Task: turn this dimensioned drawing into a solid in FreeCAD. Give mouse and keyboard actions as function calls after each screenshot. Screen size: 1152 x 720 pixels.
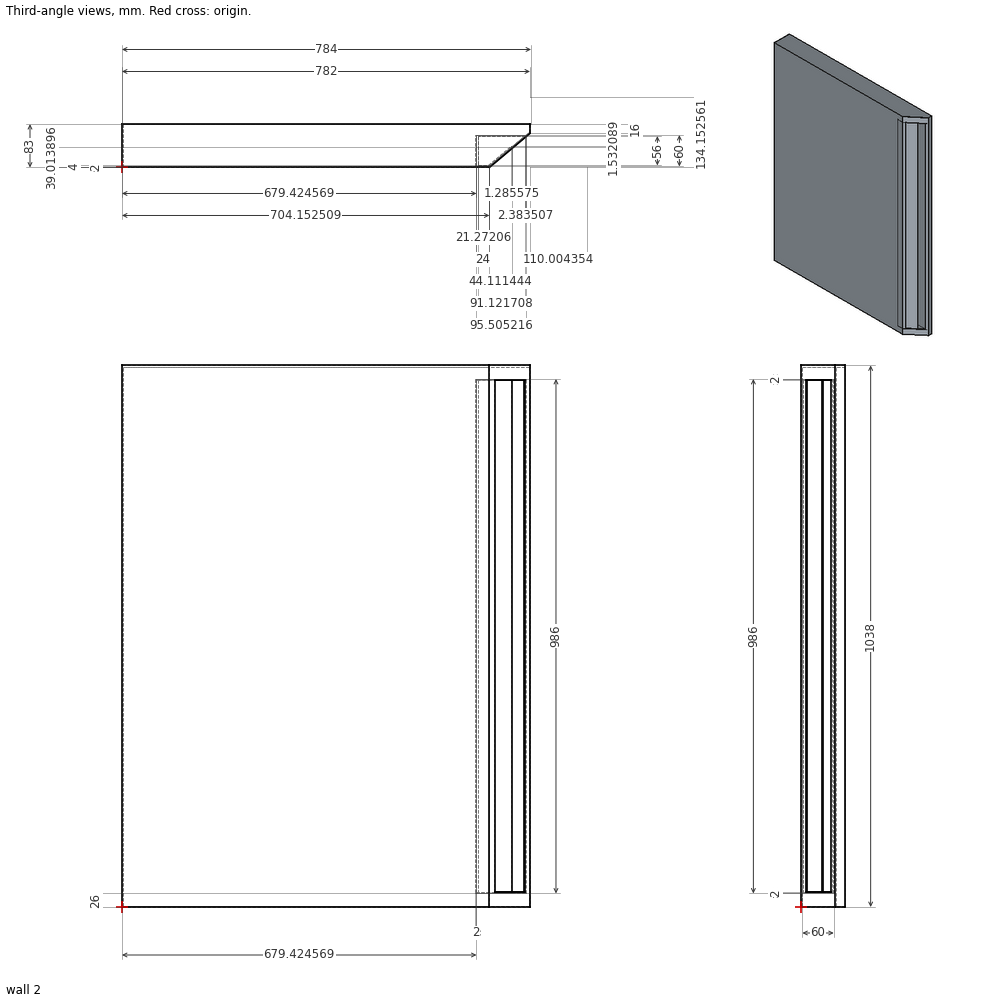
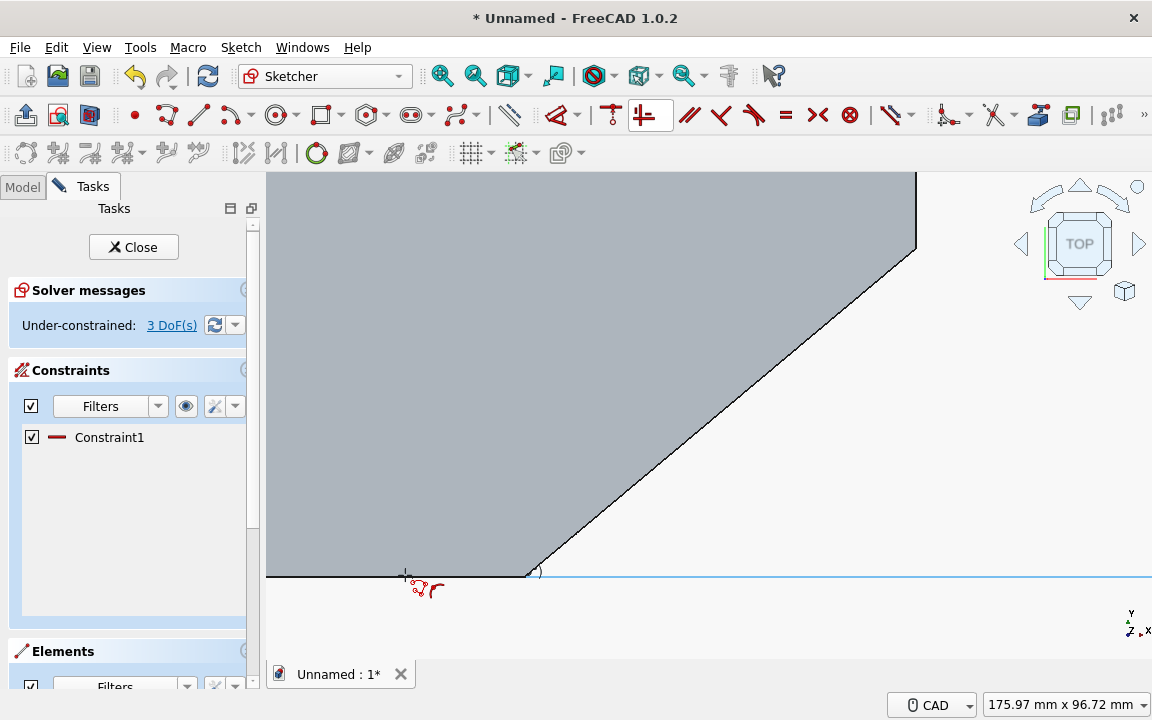
click(881, 265)
click(400, 265)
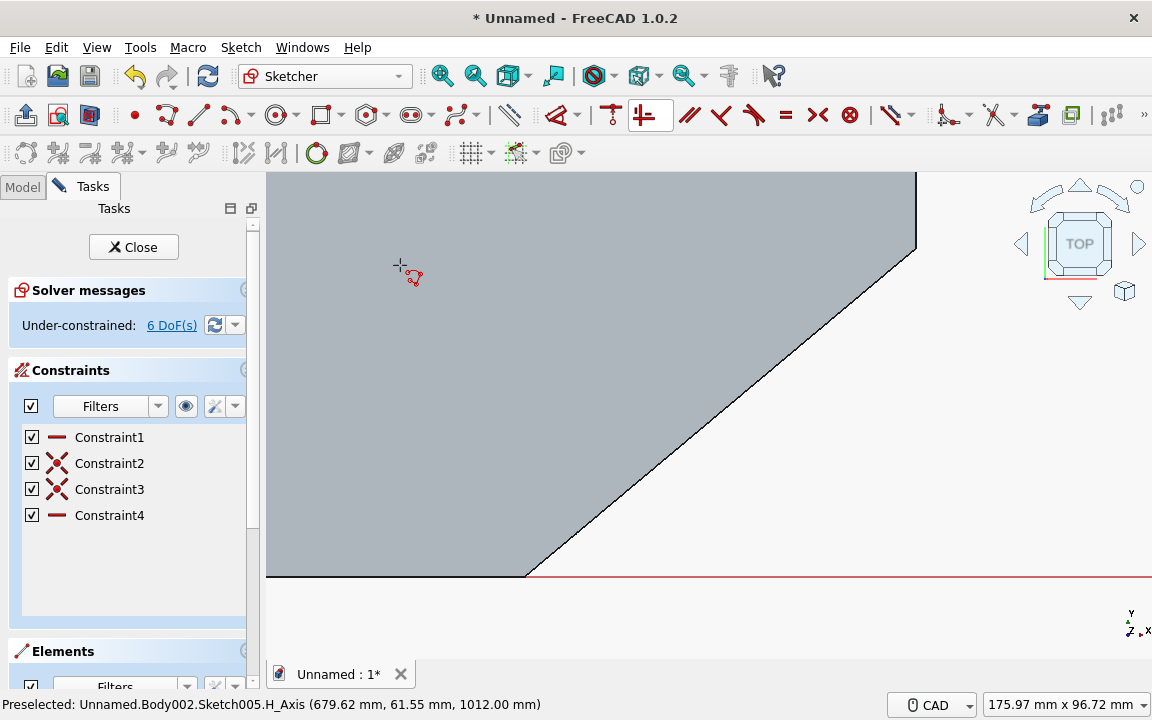
scroll(400, 567, up, 3)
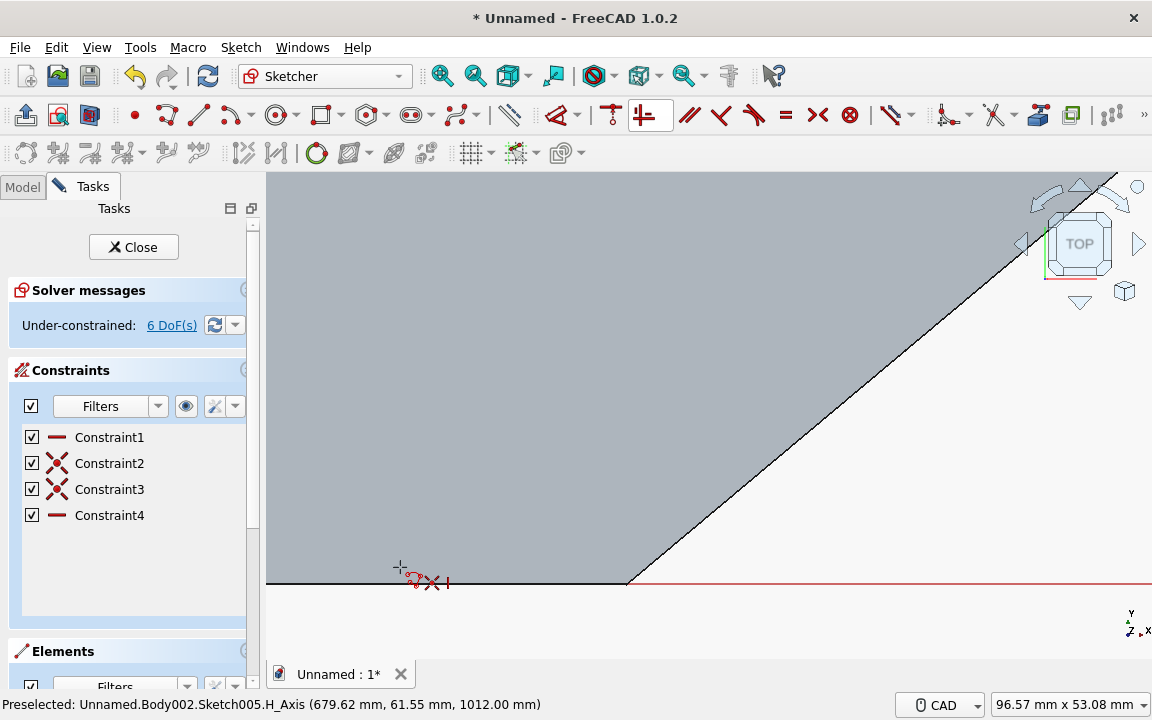
click(400, 567)
key(Escape)
key(Escape)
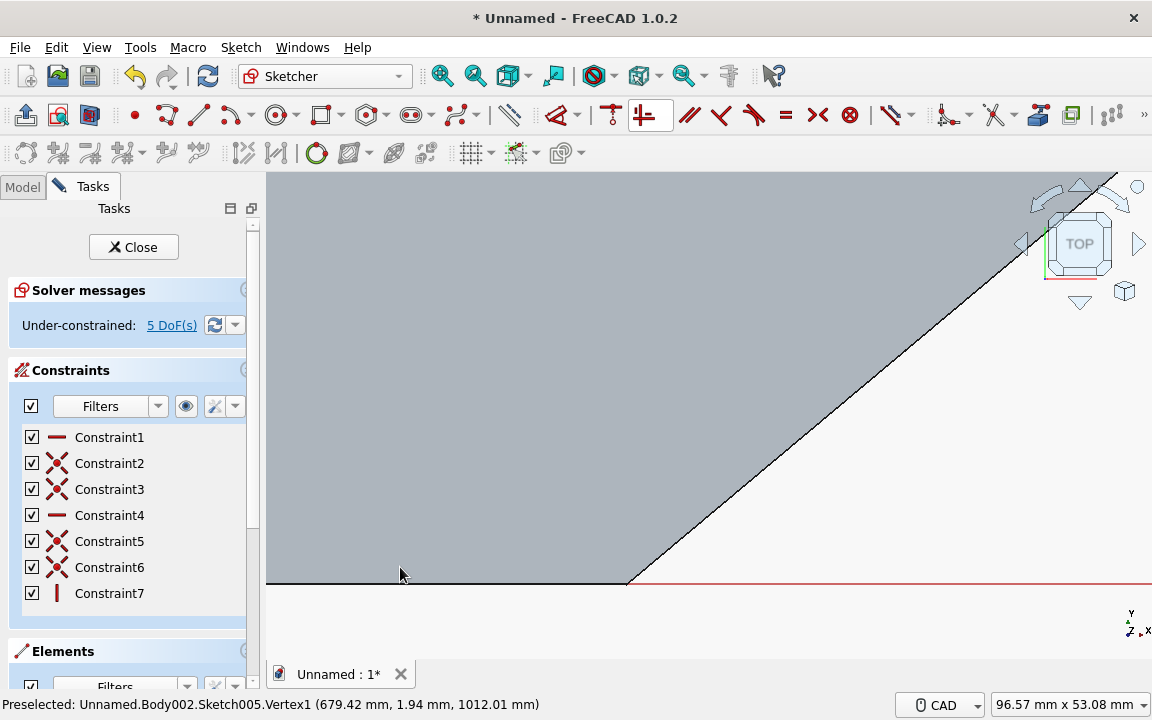
click(556, 116)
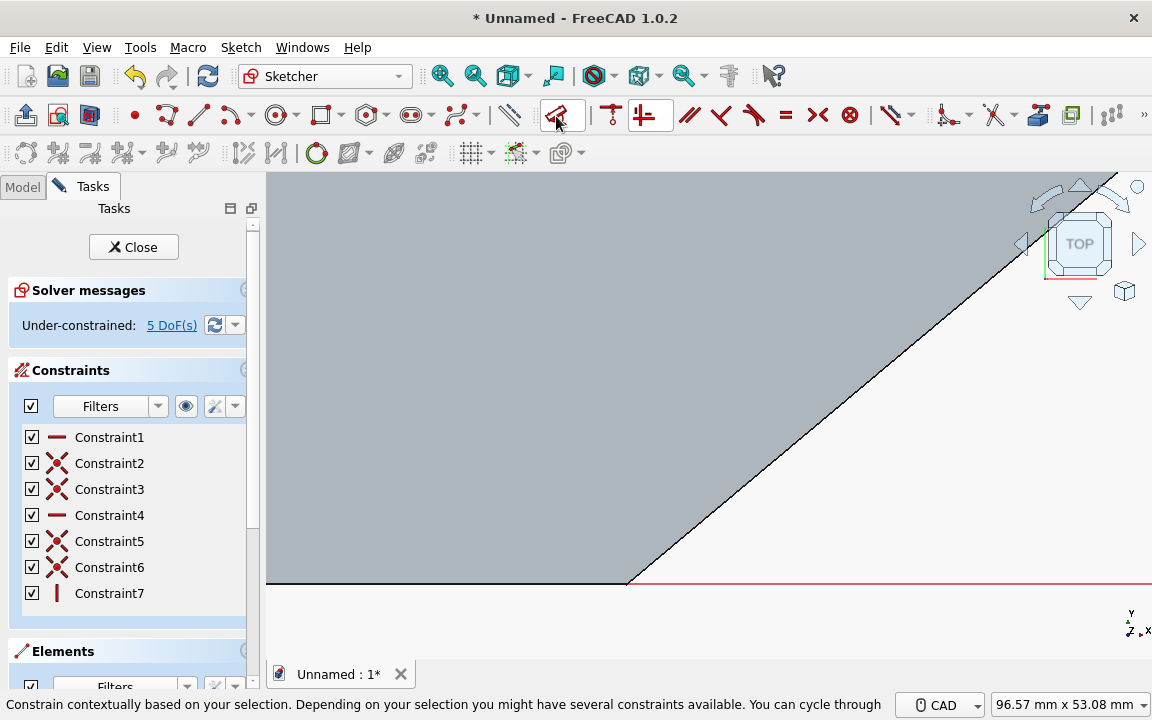
click(466, 567)
click(510, 601)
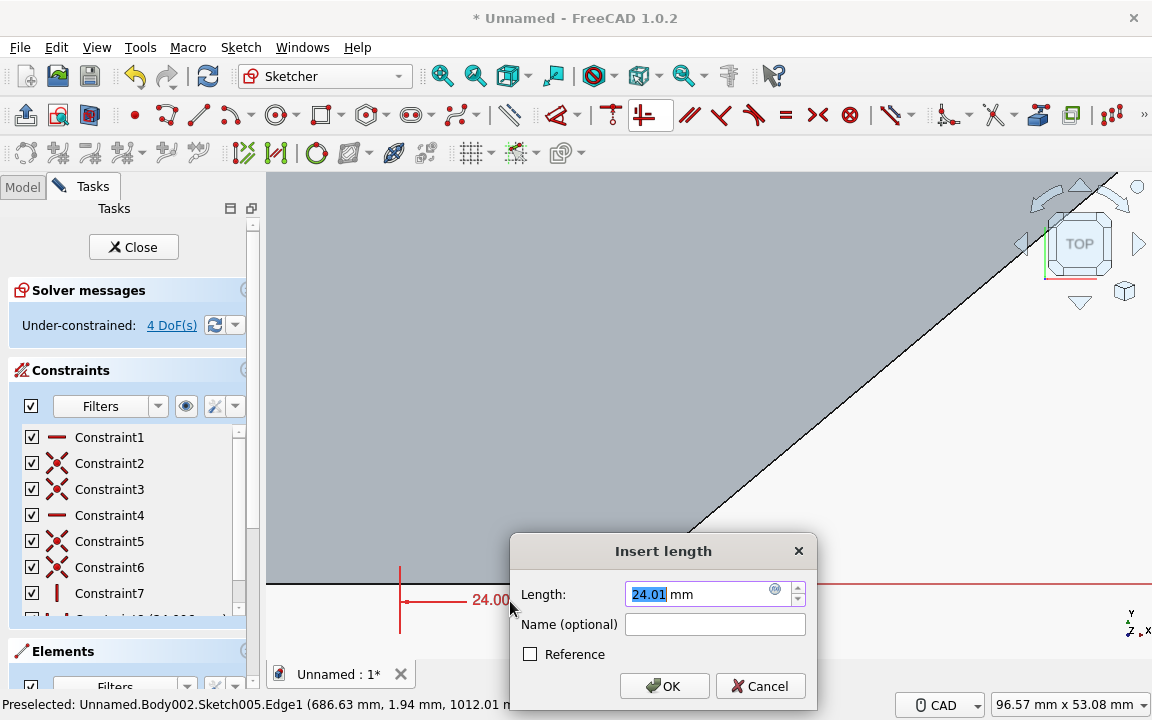
text(24)
key(Return)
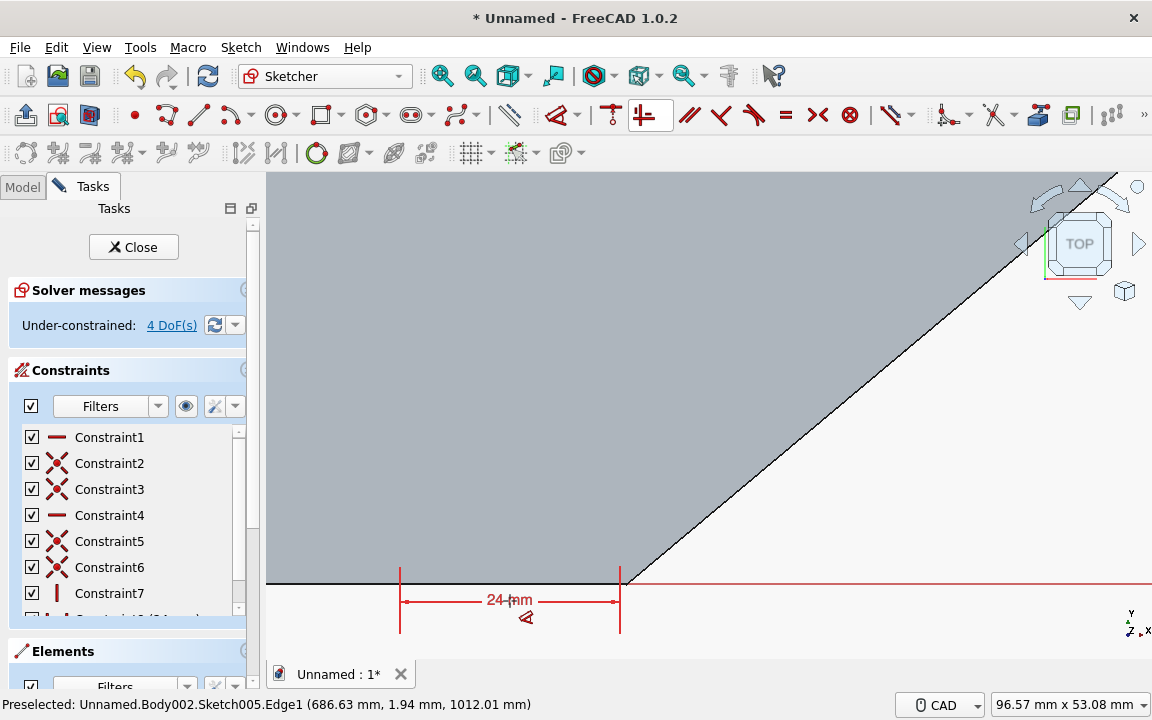
click(400, 402)
click(366, 383)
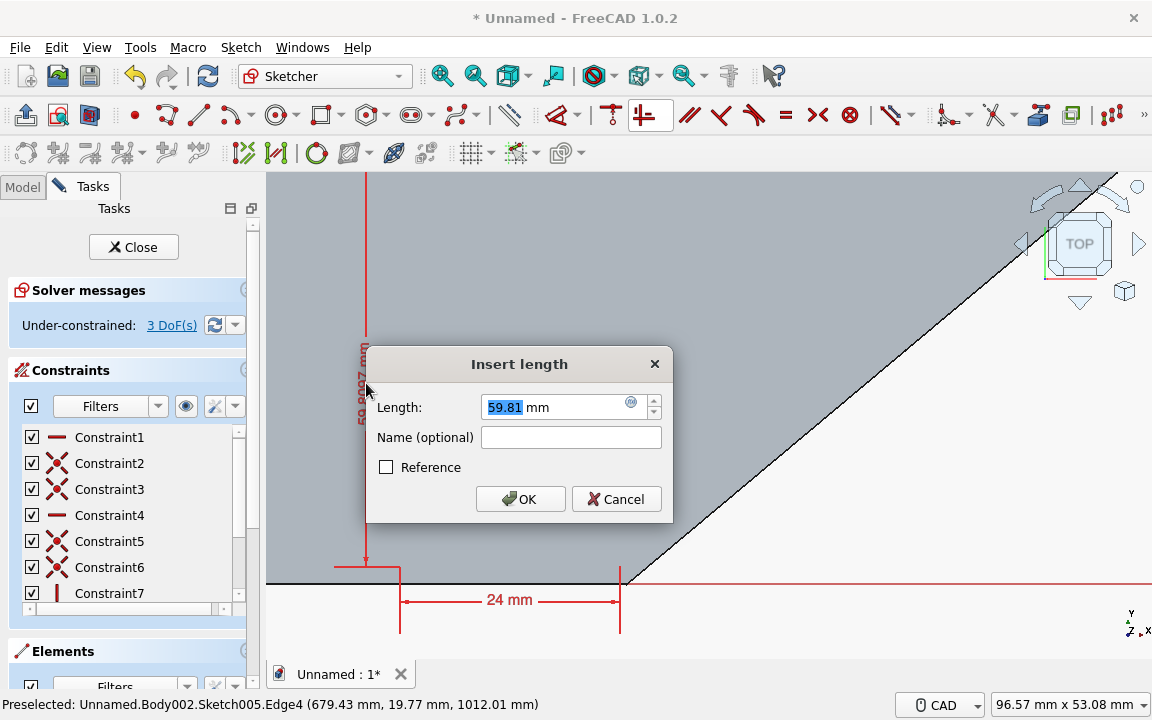
text(60)
key(Return)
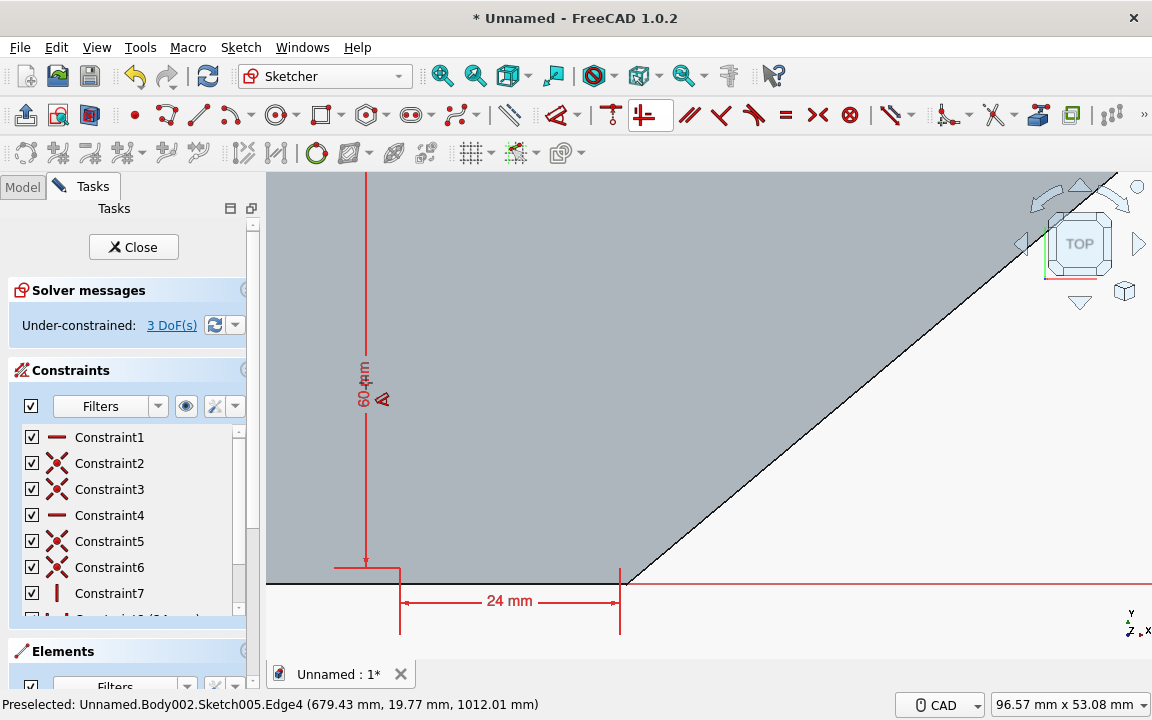
scroll(400, 568, up, 4)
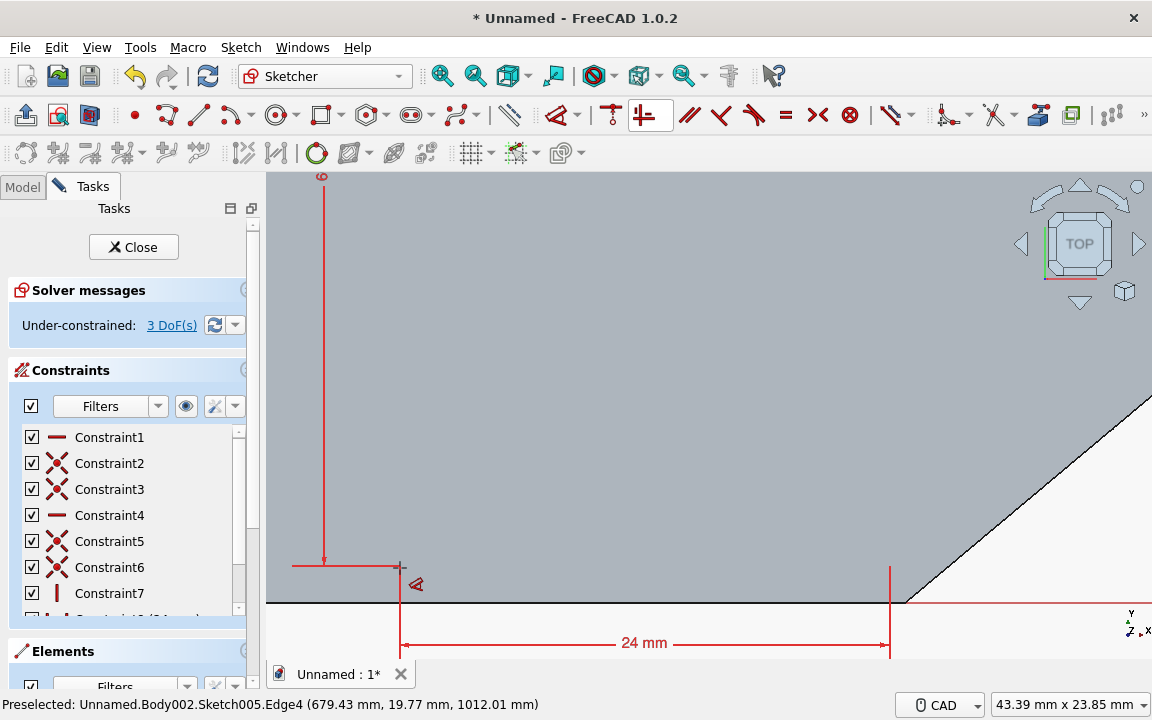
click(400, 566)
click(434, 585)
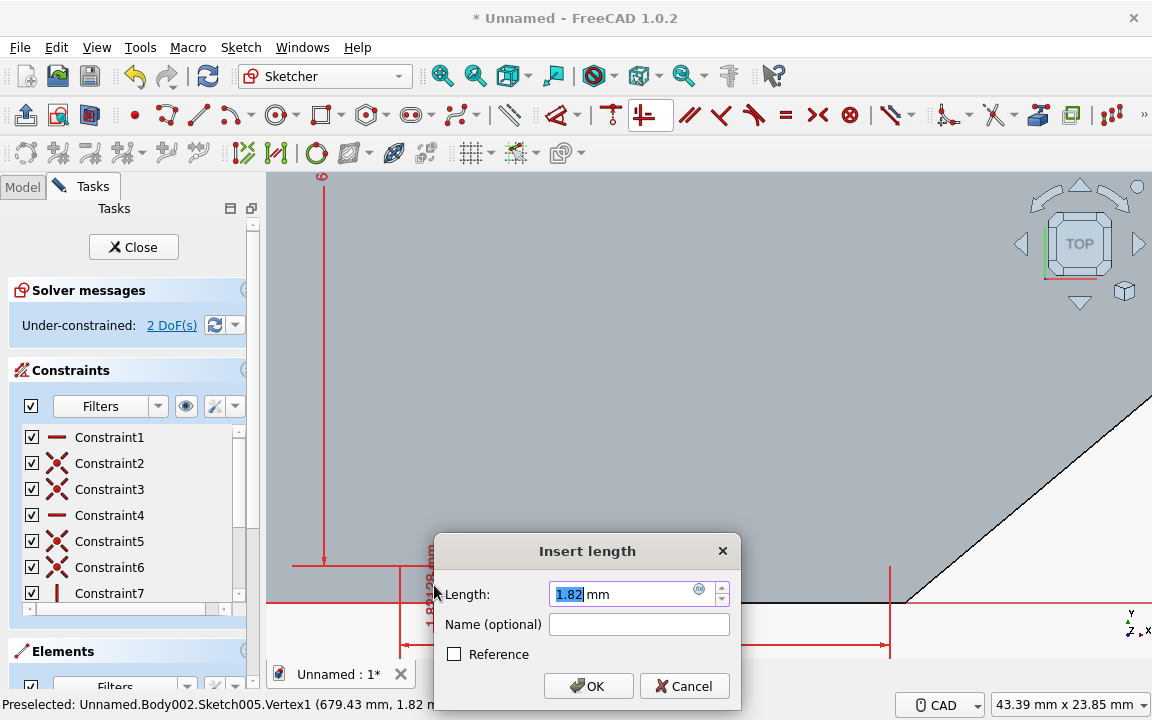
text(2)
key(Return)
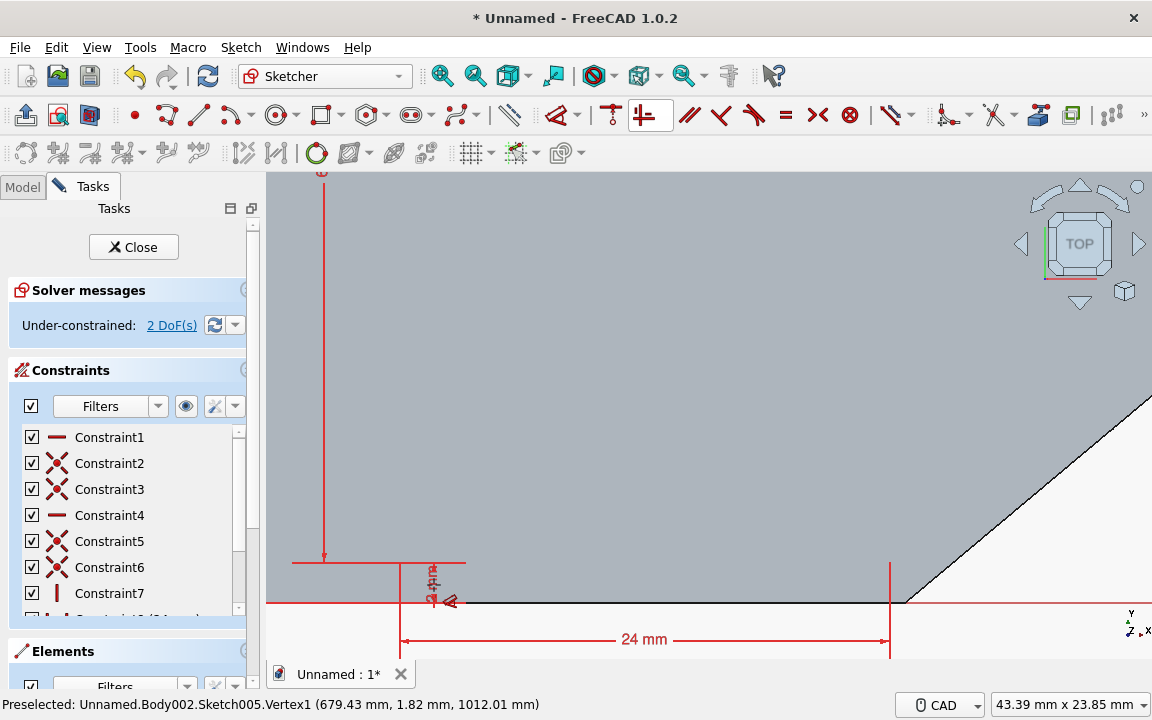
scroll(400, 568, down, 7)